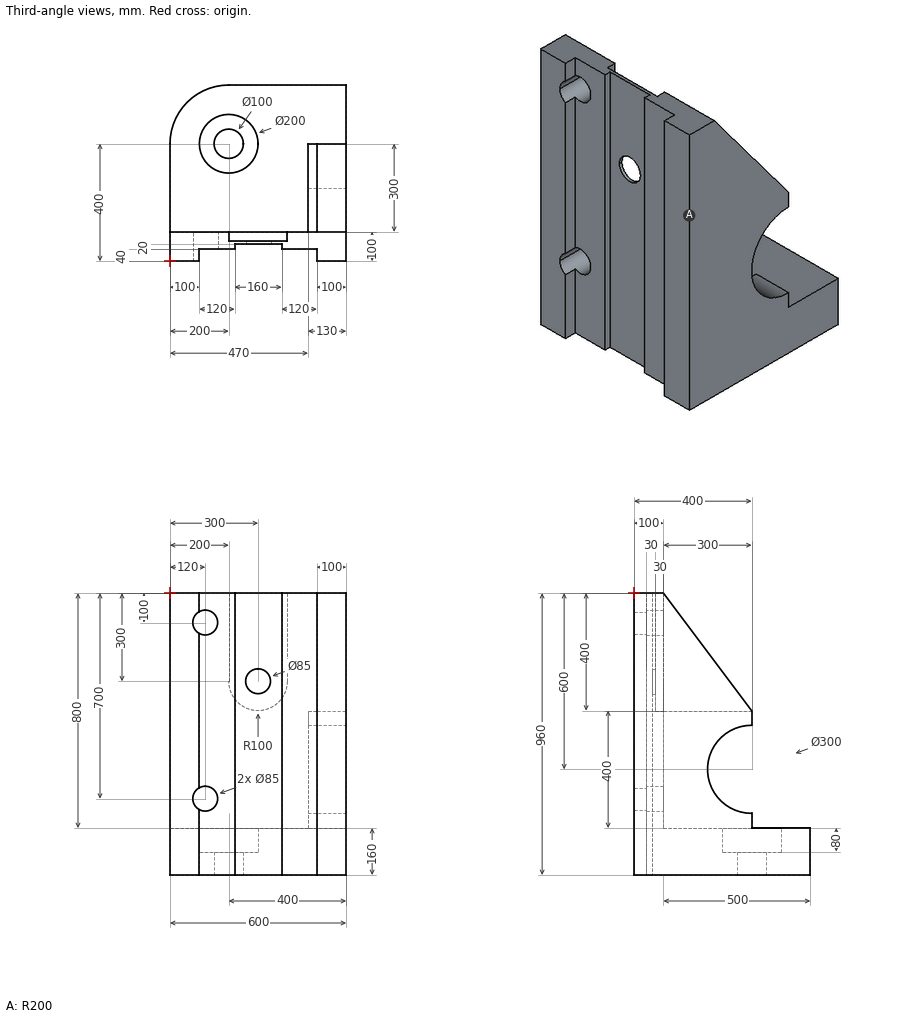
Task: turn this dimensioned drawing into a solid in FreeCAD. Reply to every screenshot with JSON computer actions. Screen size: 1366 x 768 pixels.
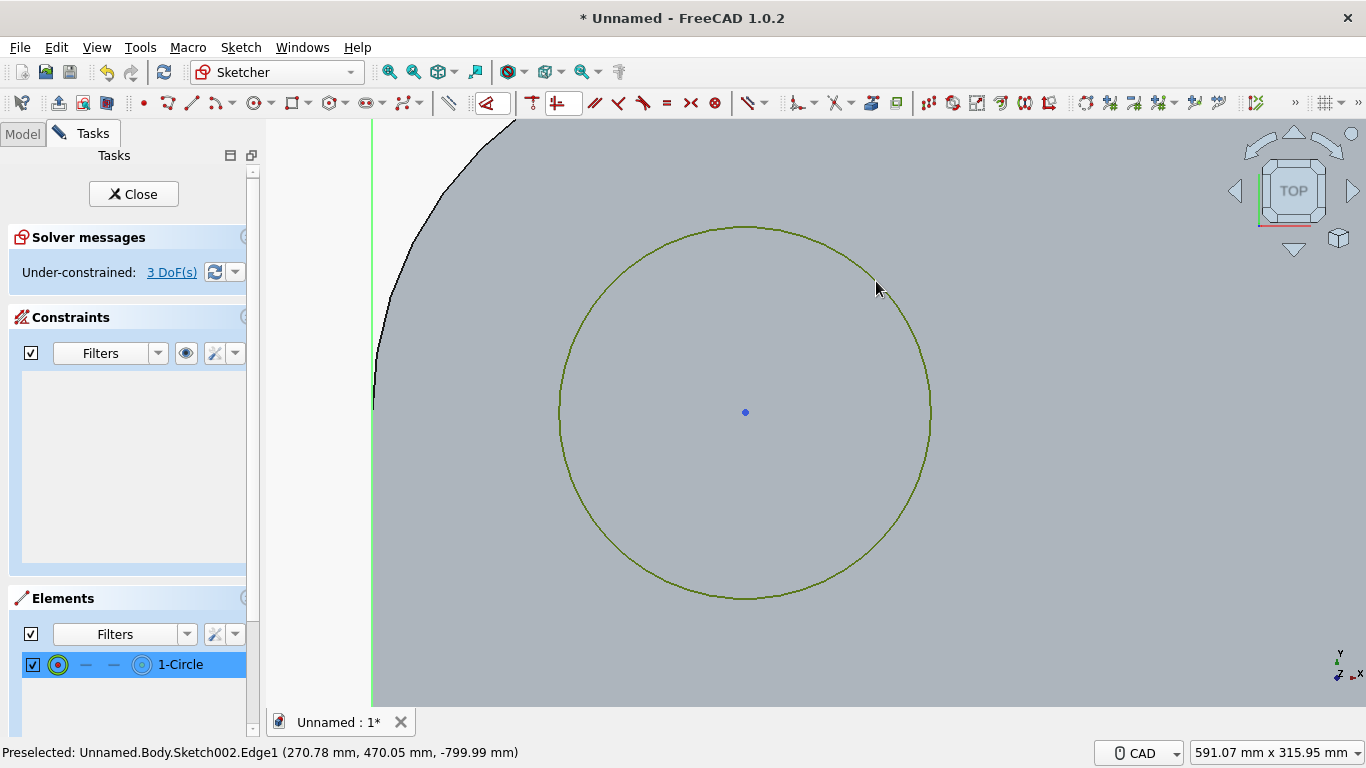
{"action": "left_click", "coordinate": [504, 104]}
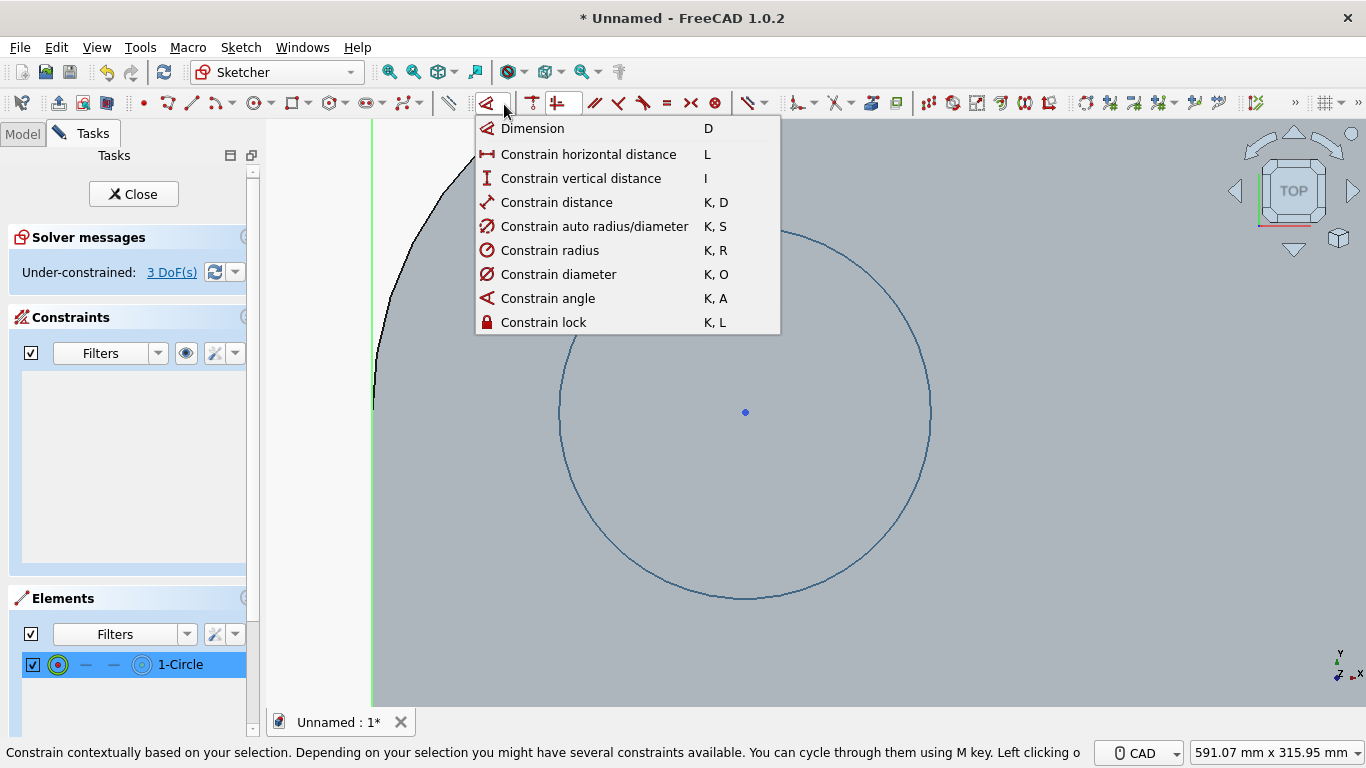
{"action": "left_click", "coordinate": [628, 274]}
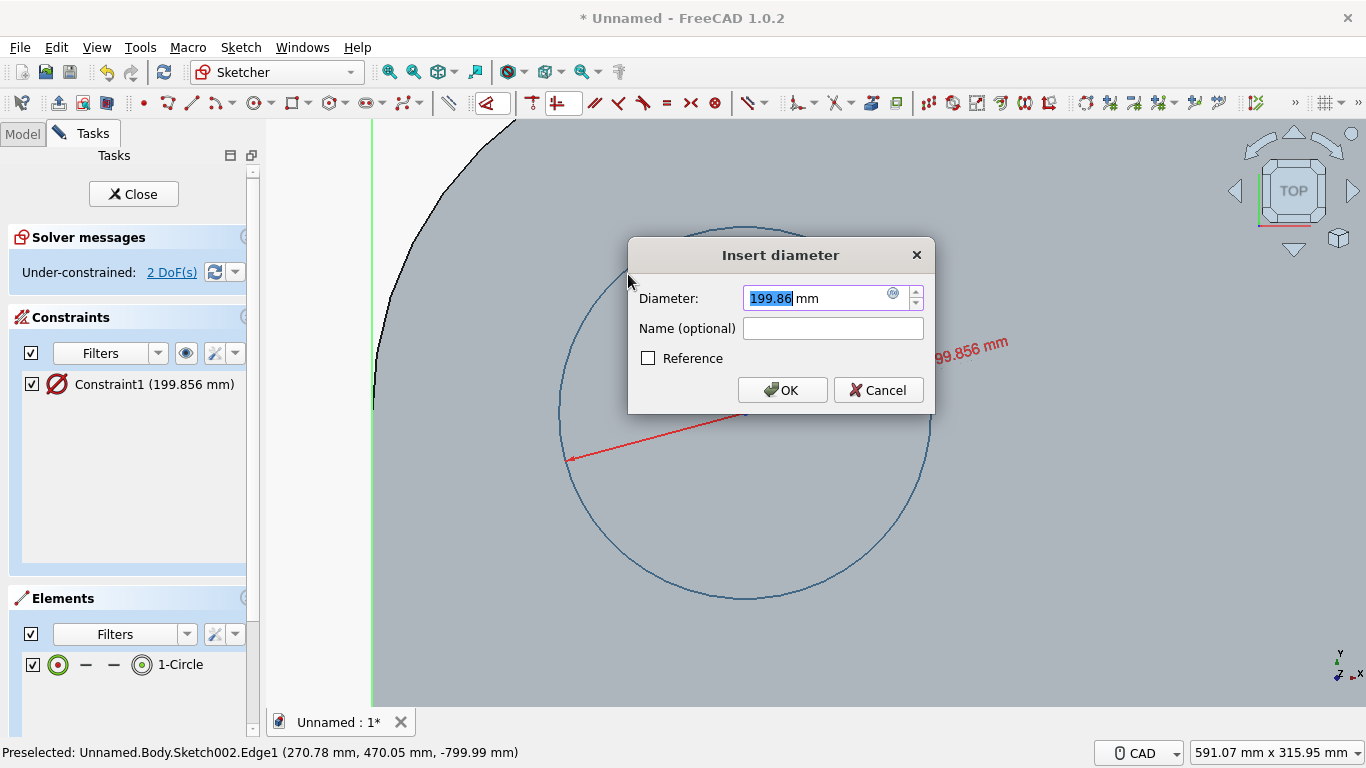
{"action": "type", "text": "200"}
{"action": "key", "text": "Return"}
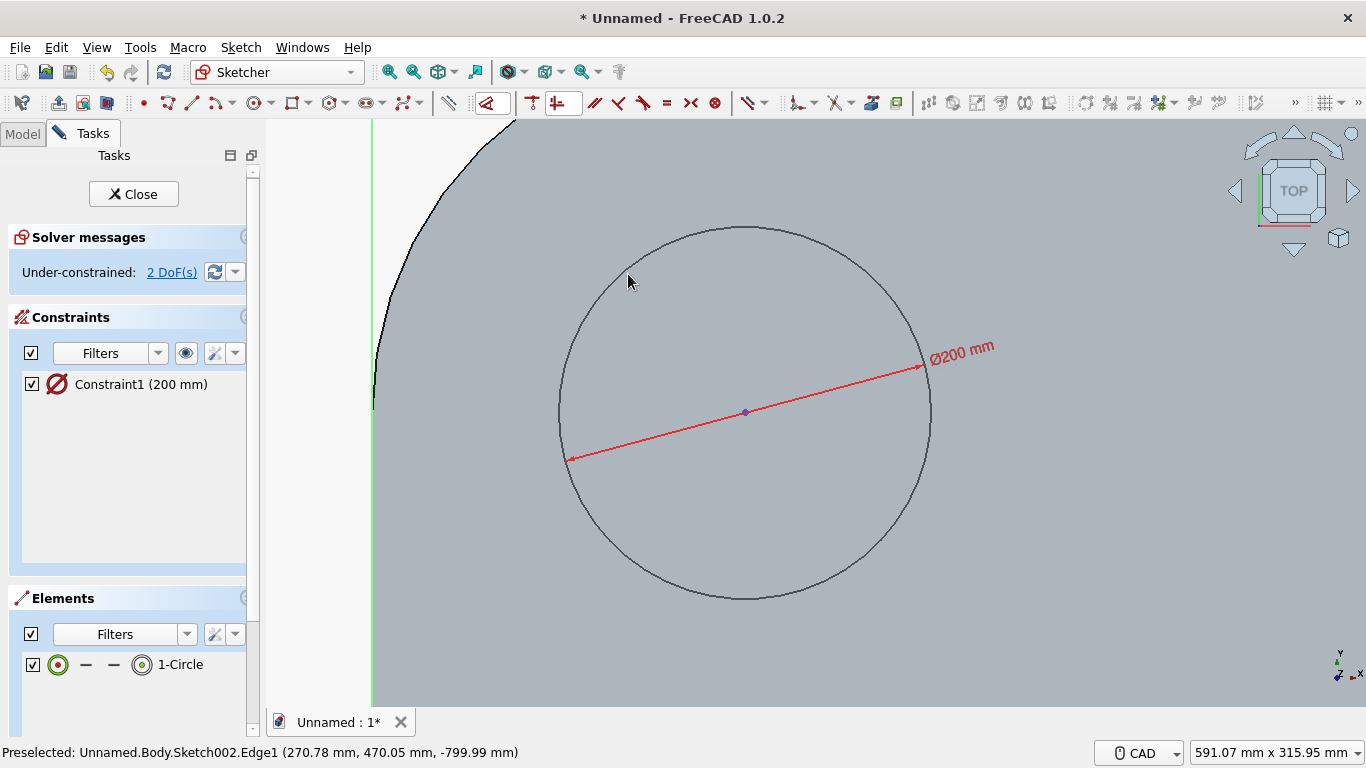
{"action": "left_click", "coordinate": [745, 413]}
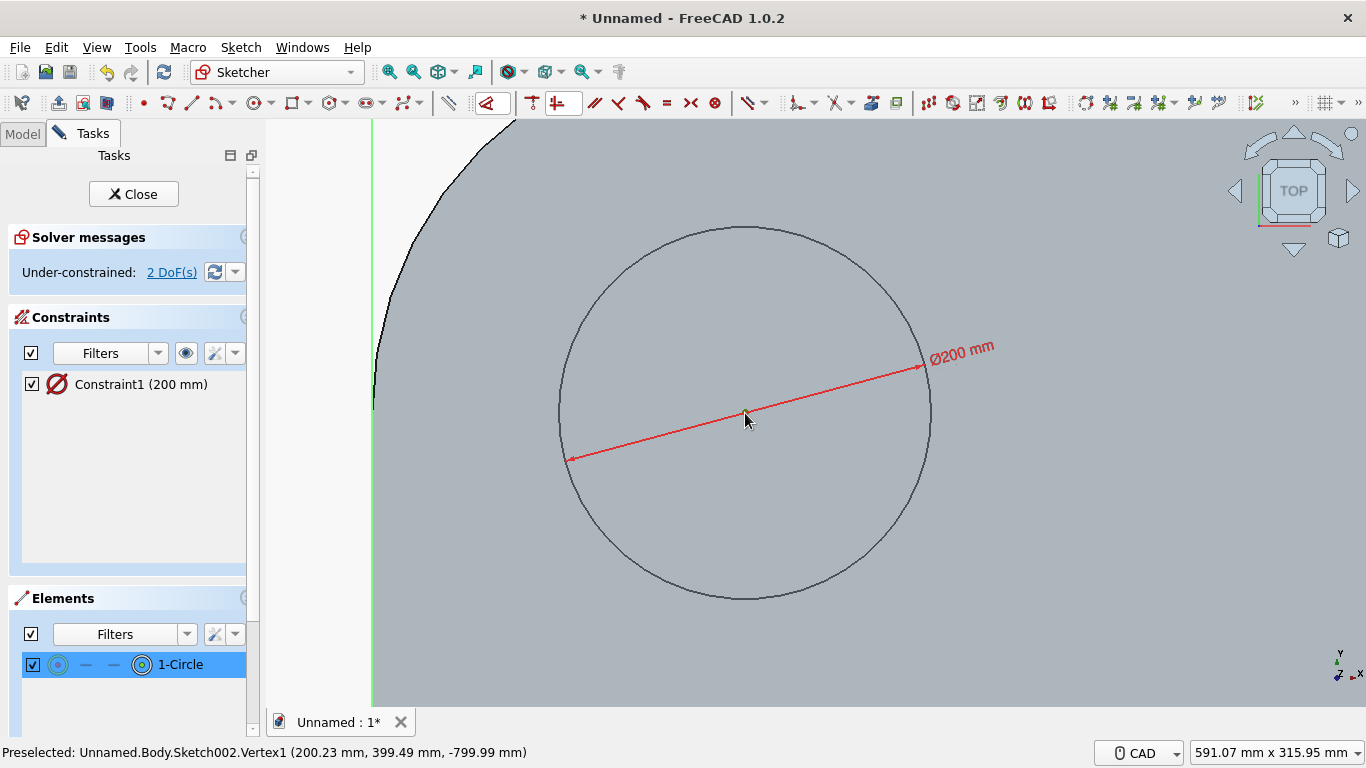
{"action": "key", "text": "l"}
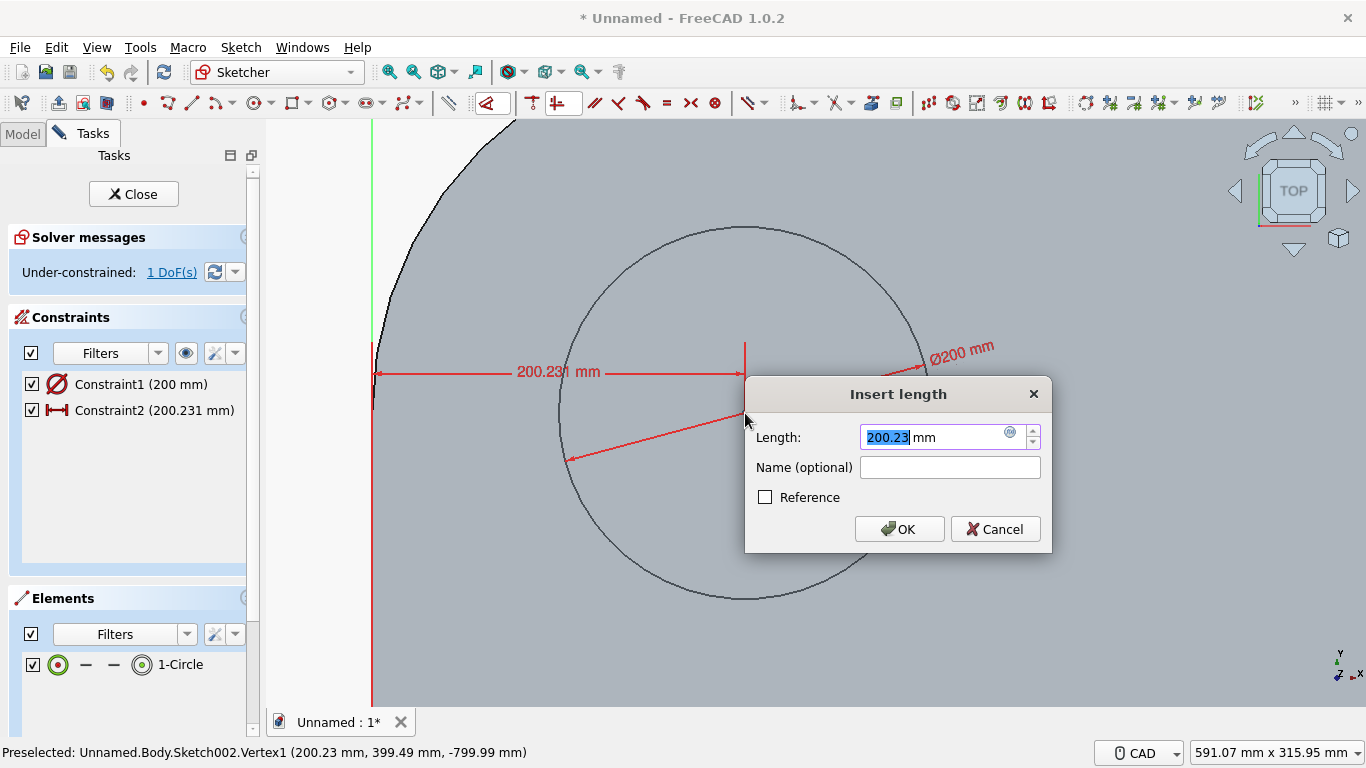
{"action": "type", "text": "200"}
{"action": "key", "text": "Return"}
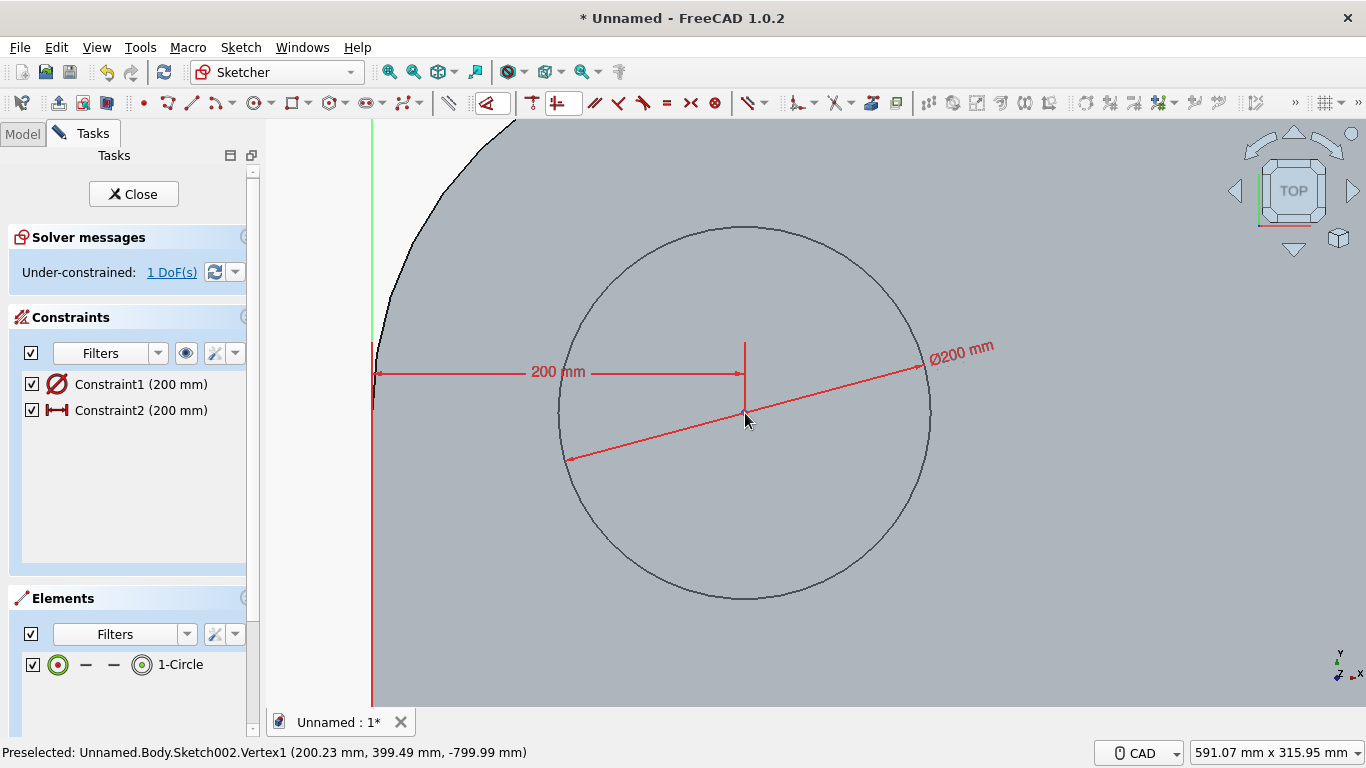
{"action": "left_click", "coordinate": [745, 413]}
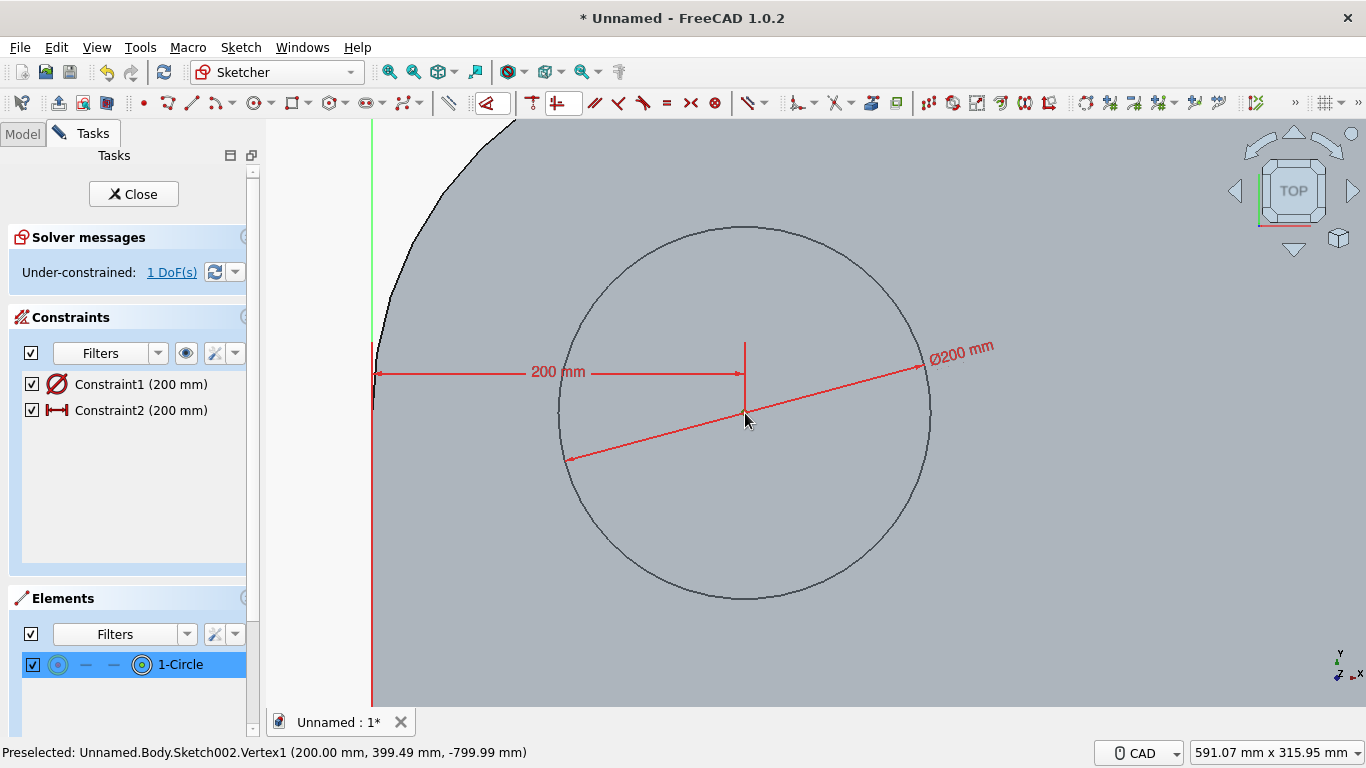
{"action": "key", "text": "i"}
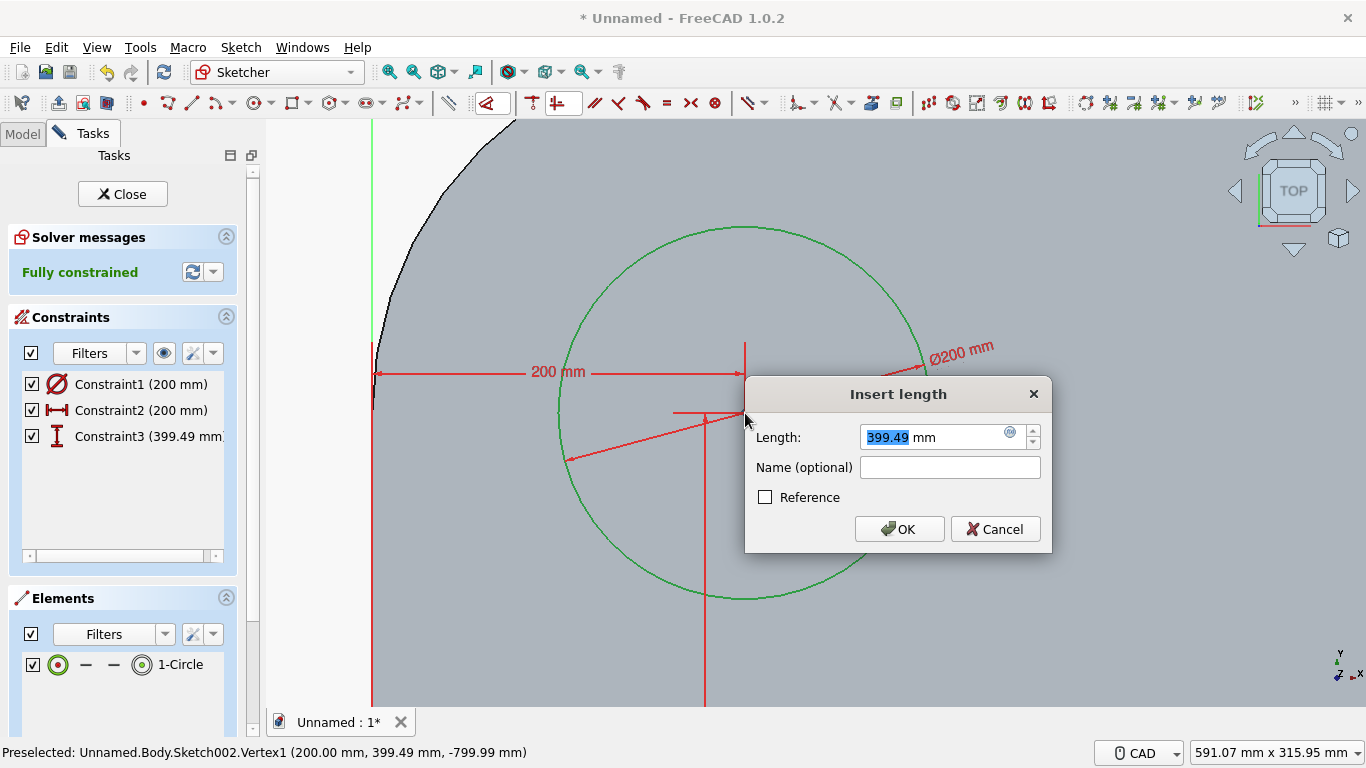
{"action": "type", "text": "400"}
{"action": "key", "text": "Return"}